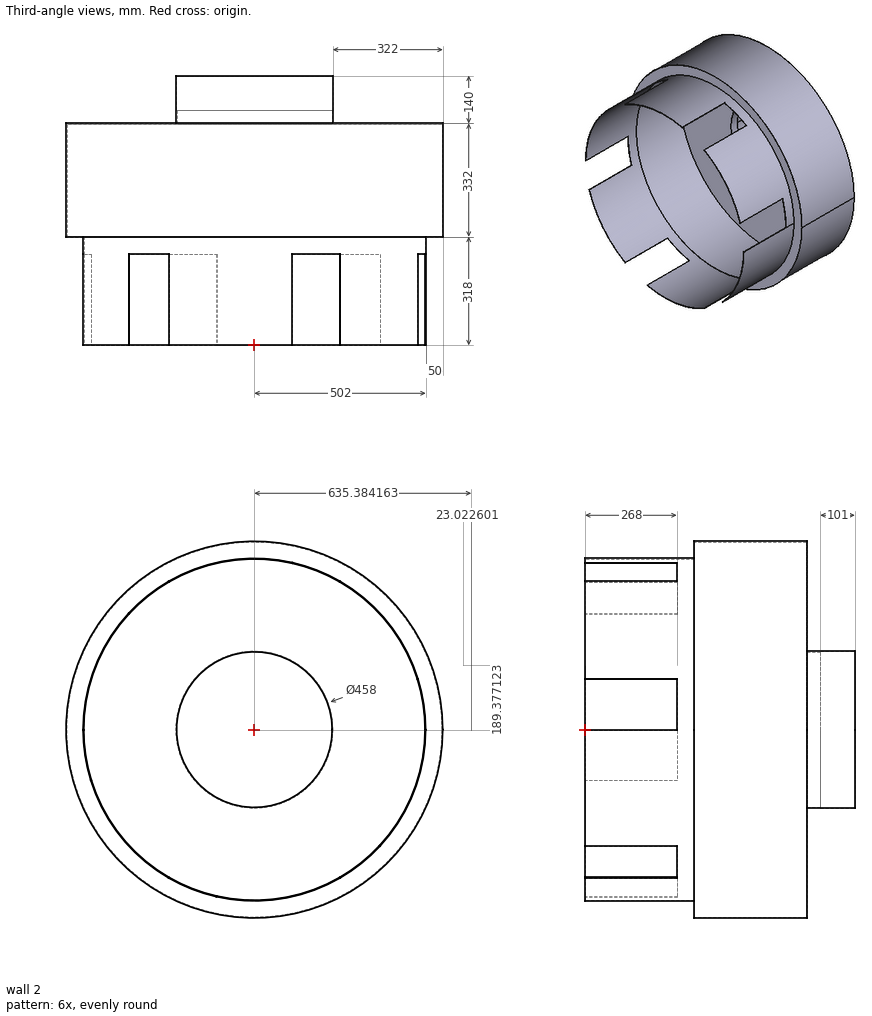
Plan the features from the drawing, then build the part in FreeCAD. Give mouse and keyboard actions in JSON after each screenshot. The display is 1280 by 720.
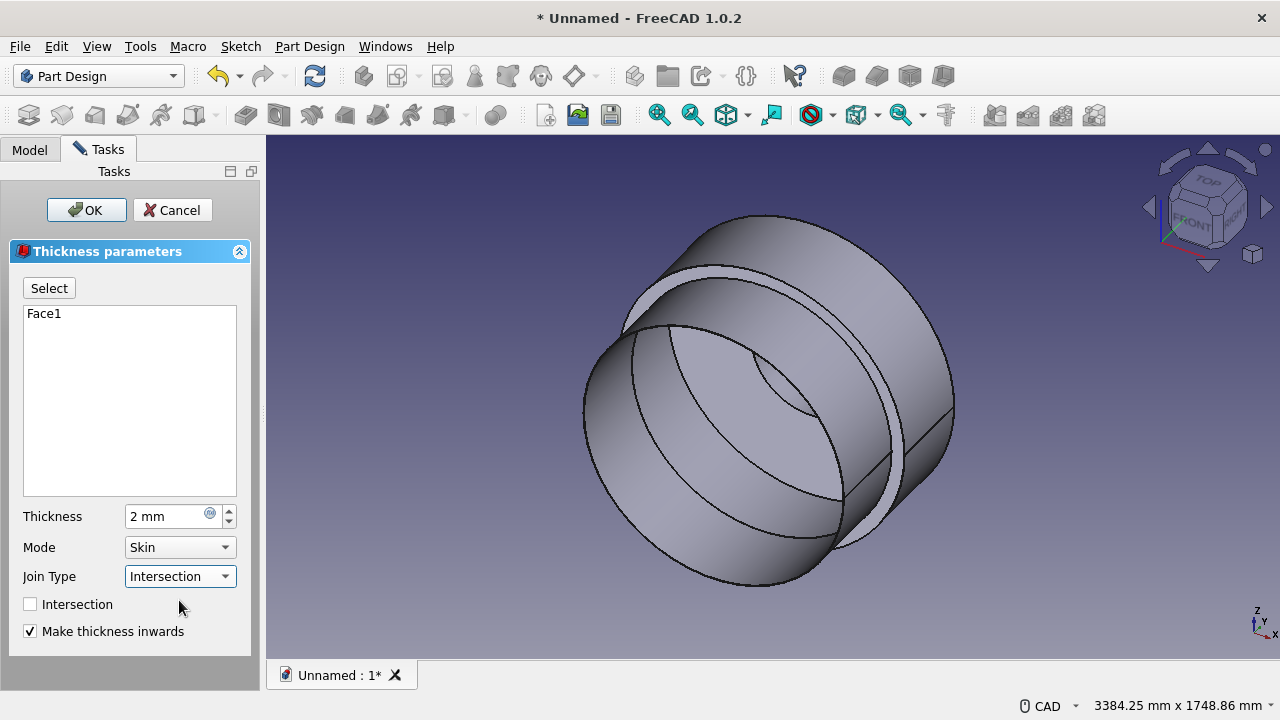
{"action": "left_click", "coordinate": [87, 210]}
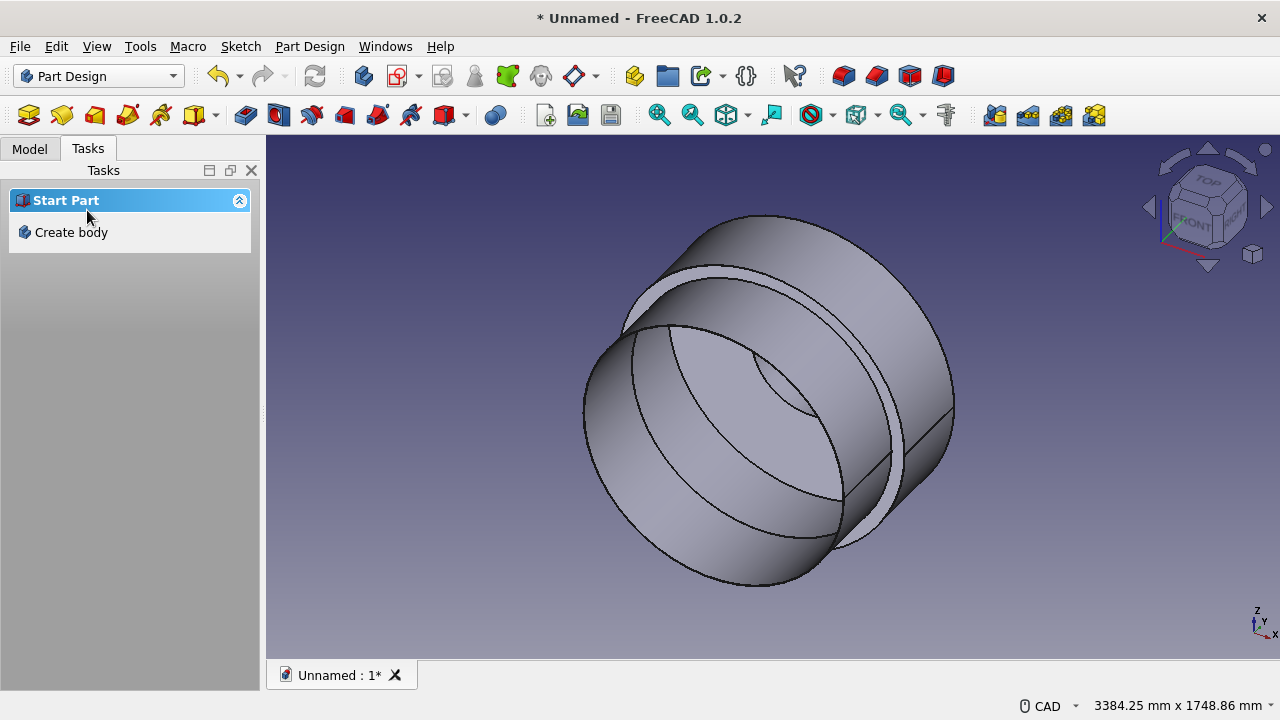
{"action": "key", "text": "4"}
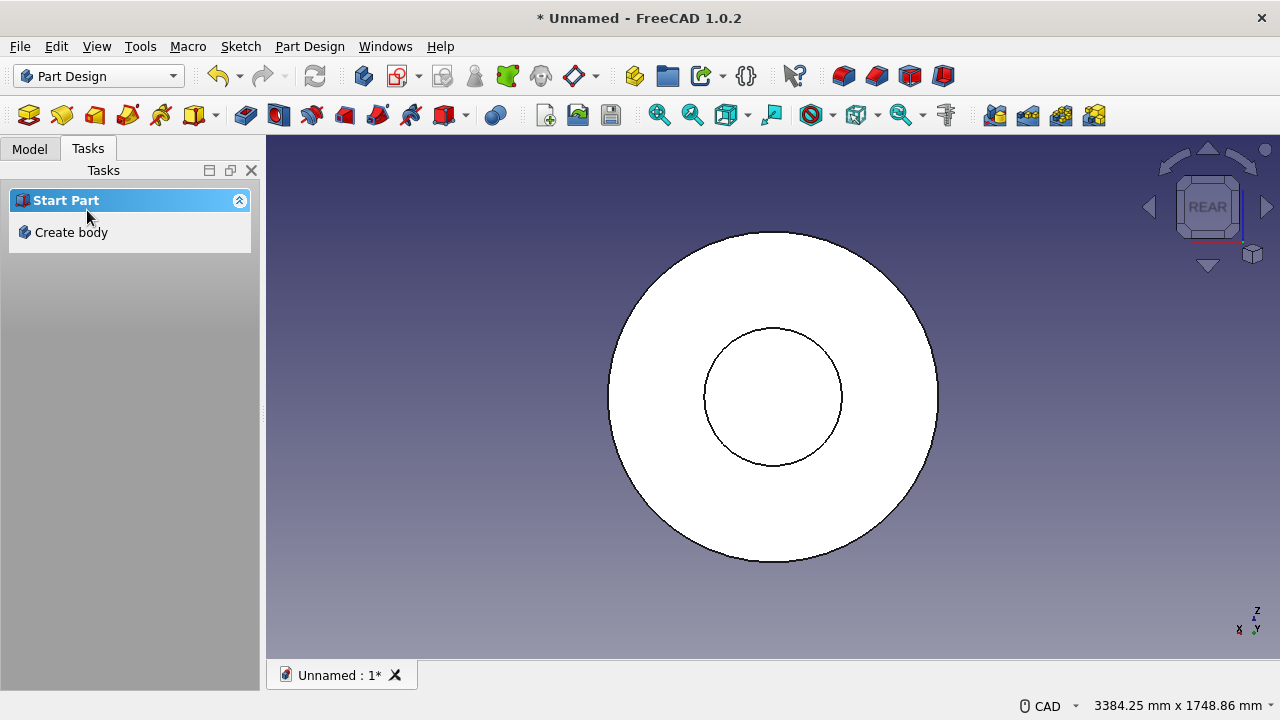
{"action": "left_click", "coordinate": [773, 396]}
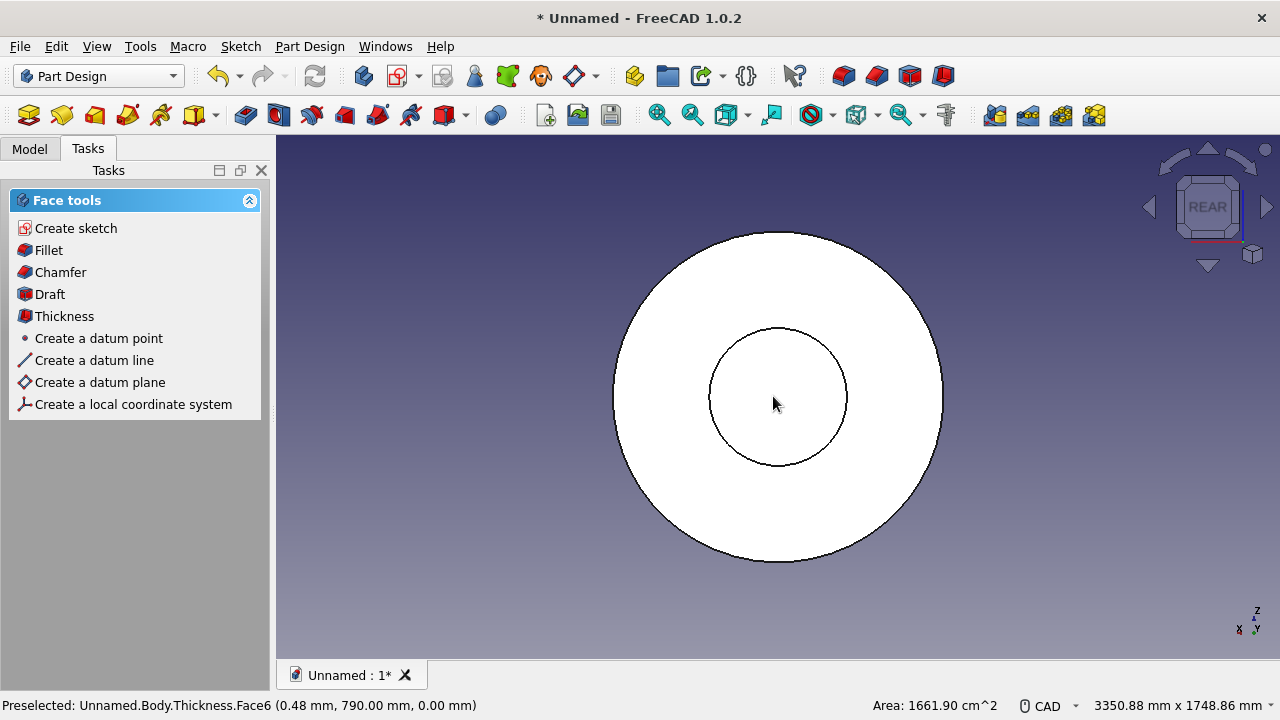
{"action": "left_click", "coordinate": [396, 76]}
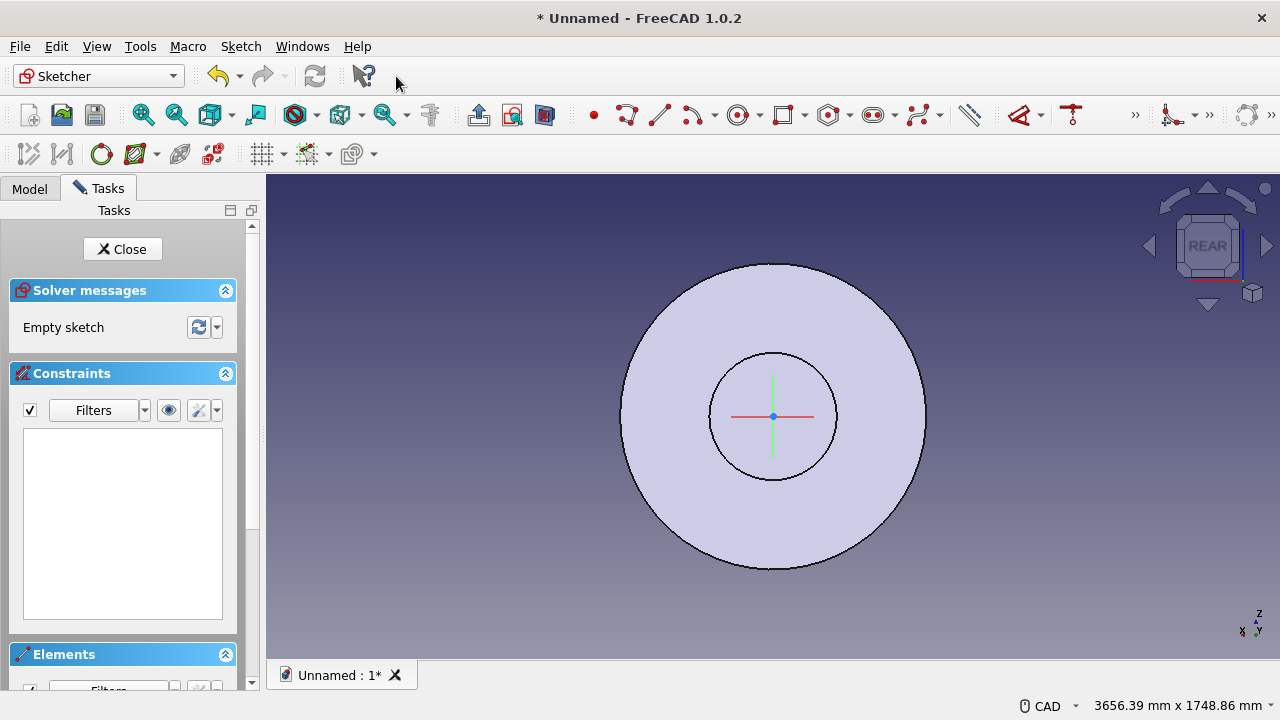
{"action": "scroll", "coordinate": [829, 416], "scroll_direction": "up", "scroll_amount": 4}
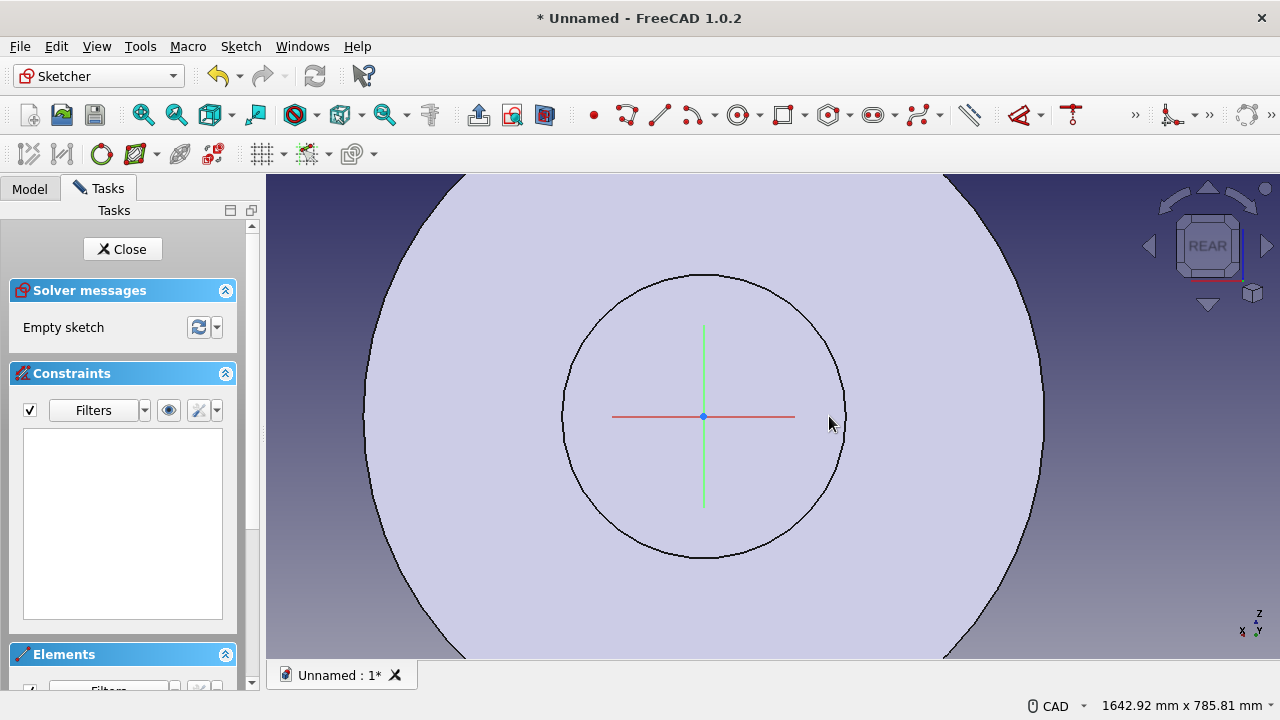
{"action": "key", "text": "g c"}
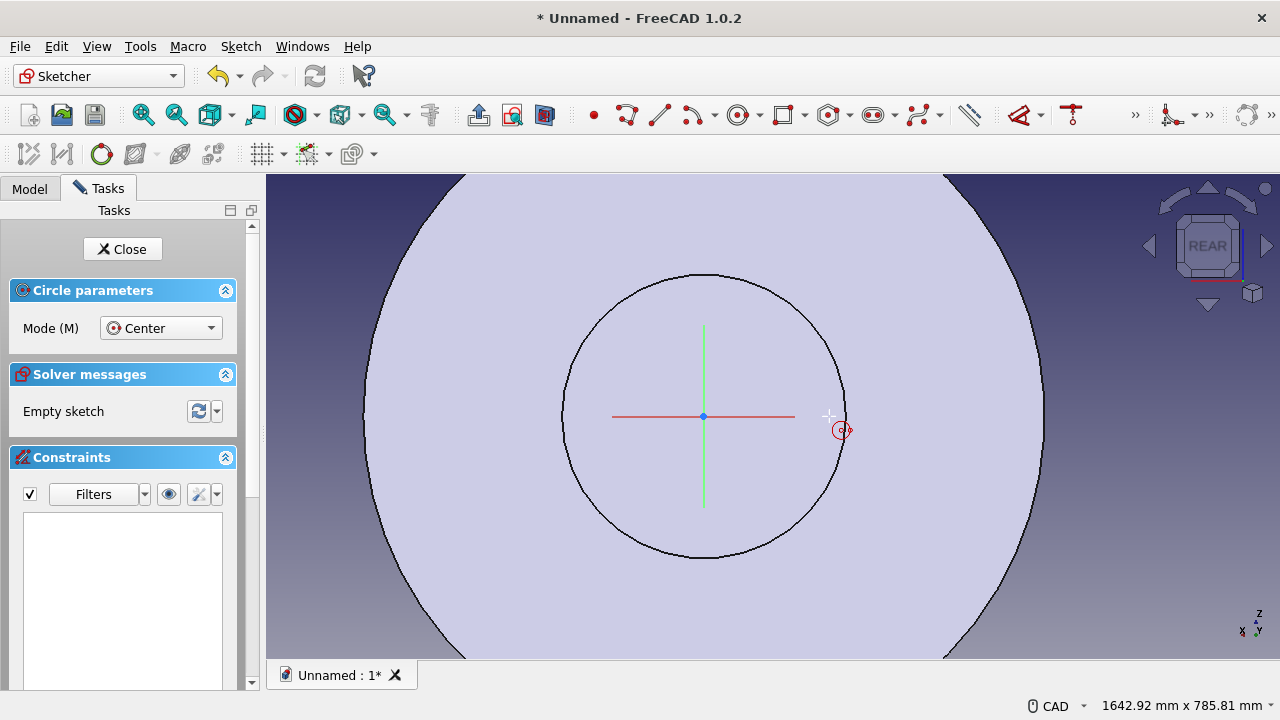
{"action": "left_click", "coordinate": [704, 416]}
{"action": "left_click", "coordinate": [804, 317]}
{"action": "key", "text": "Escape"}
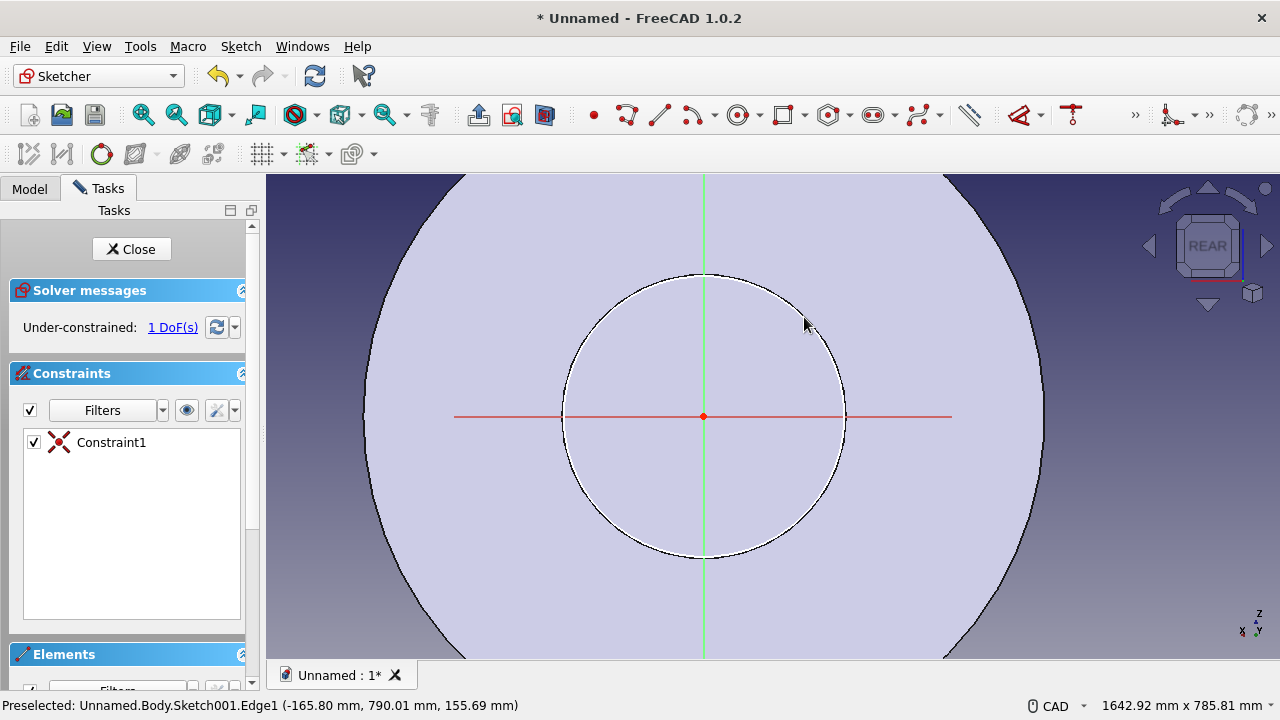
{"action": "left_click", "coordinate": [1018, 116]}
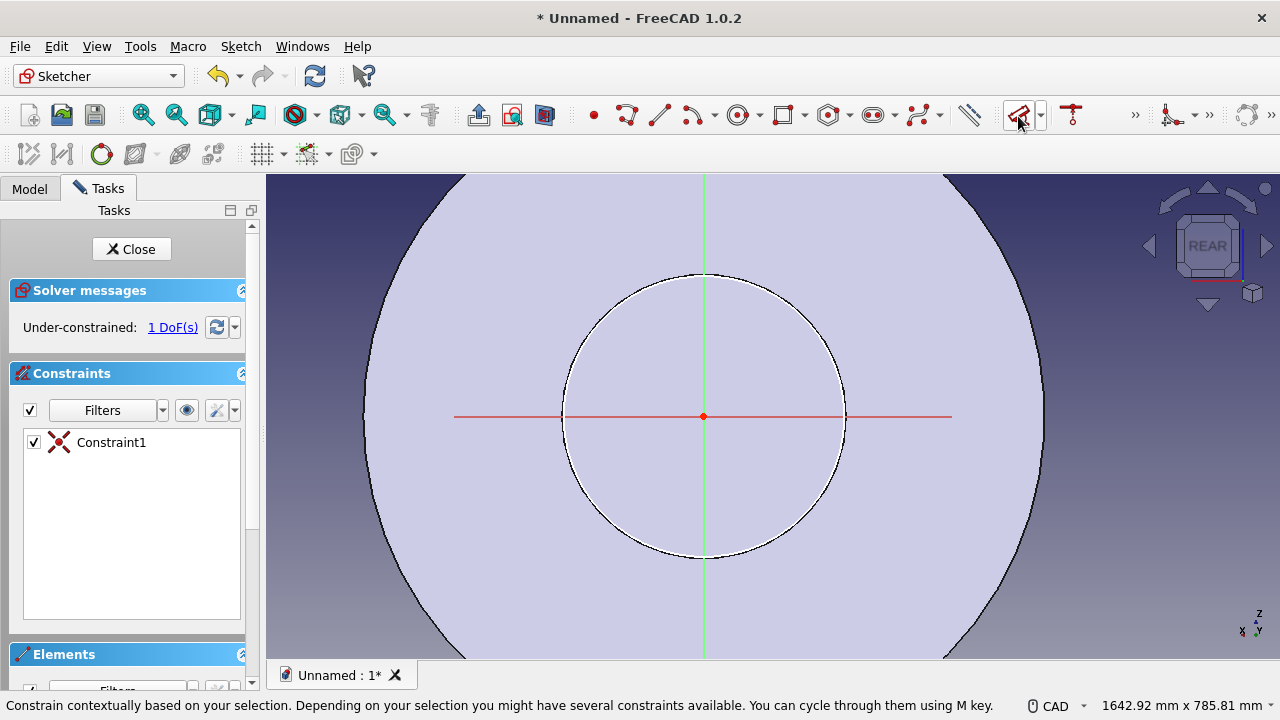
{"action": "left_click", "coordinate": [803, 317]}
{"action": "left_click", "coordinate": [826, 294]}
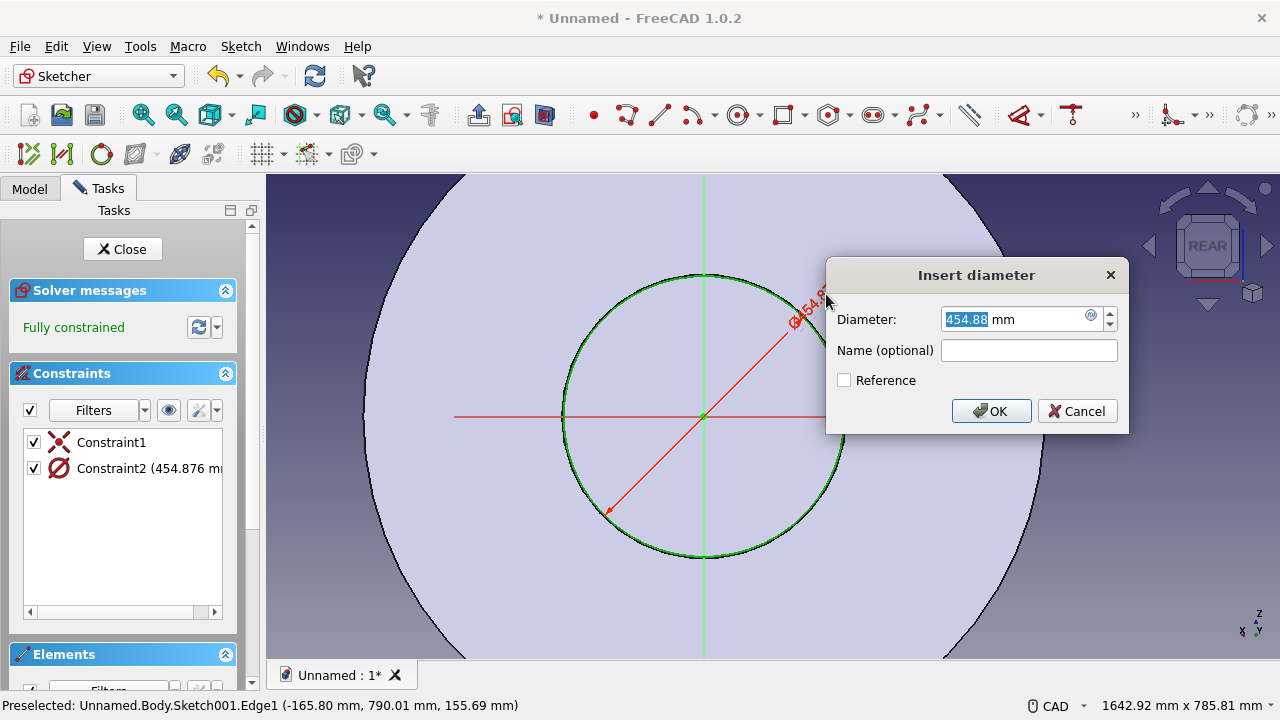
{"action": "type", "text": "458"}
{"action": "key", "text": "Return"}
{"action": "key", "text": "Escape"}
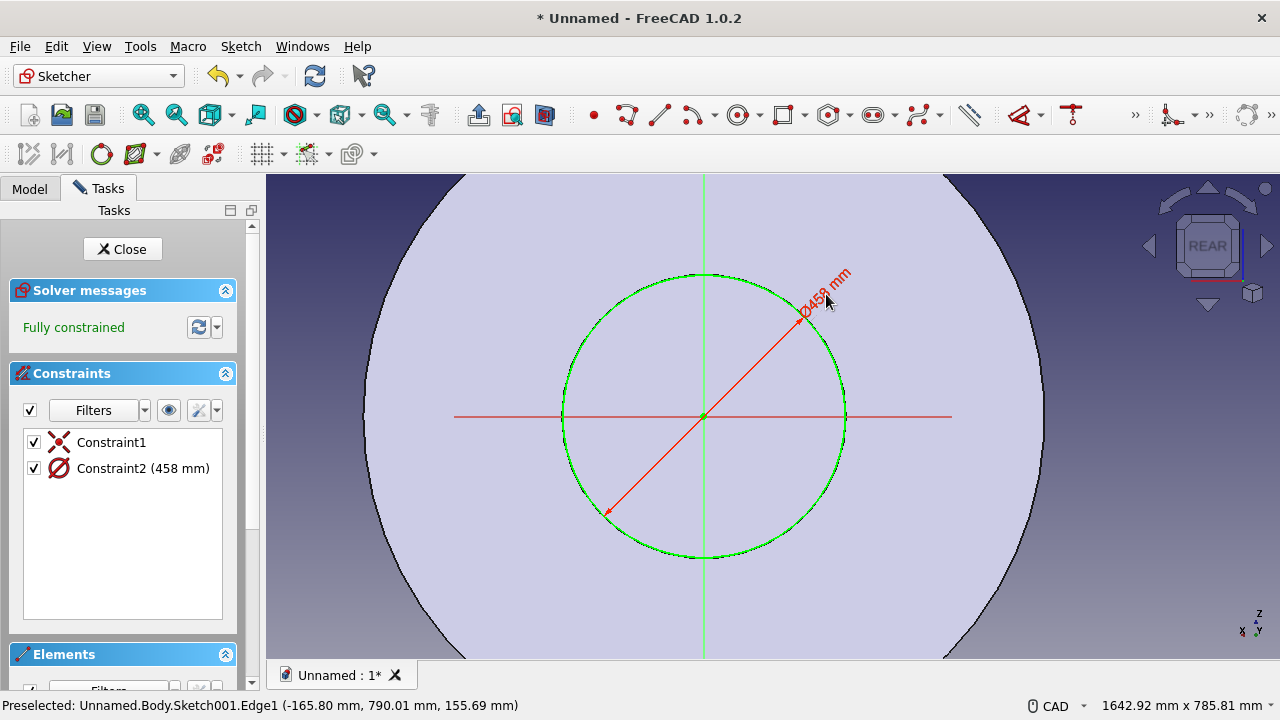
{"action": "left_click", "coordinate": [123, 249]}